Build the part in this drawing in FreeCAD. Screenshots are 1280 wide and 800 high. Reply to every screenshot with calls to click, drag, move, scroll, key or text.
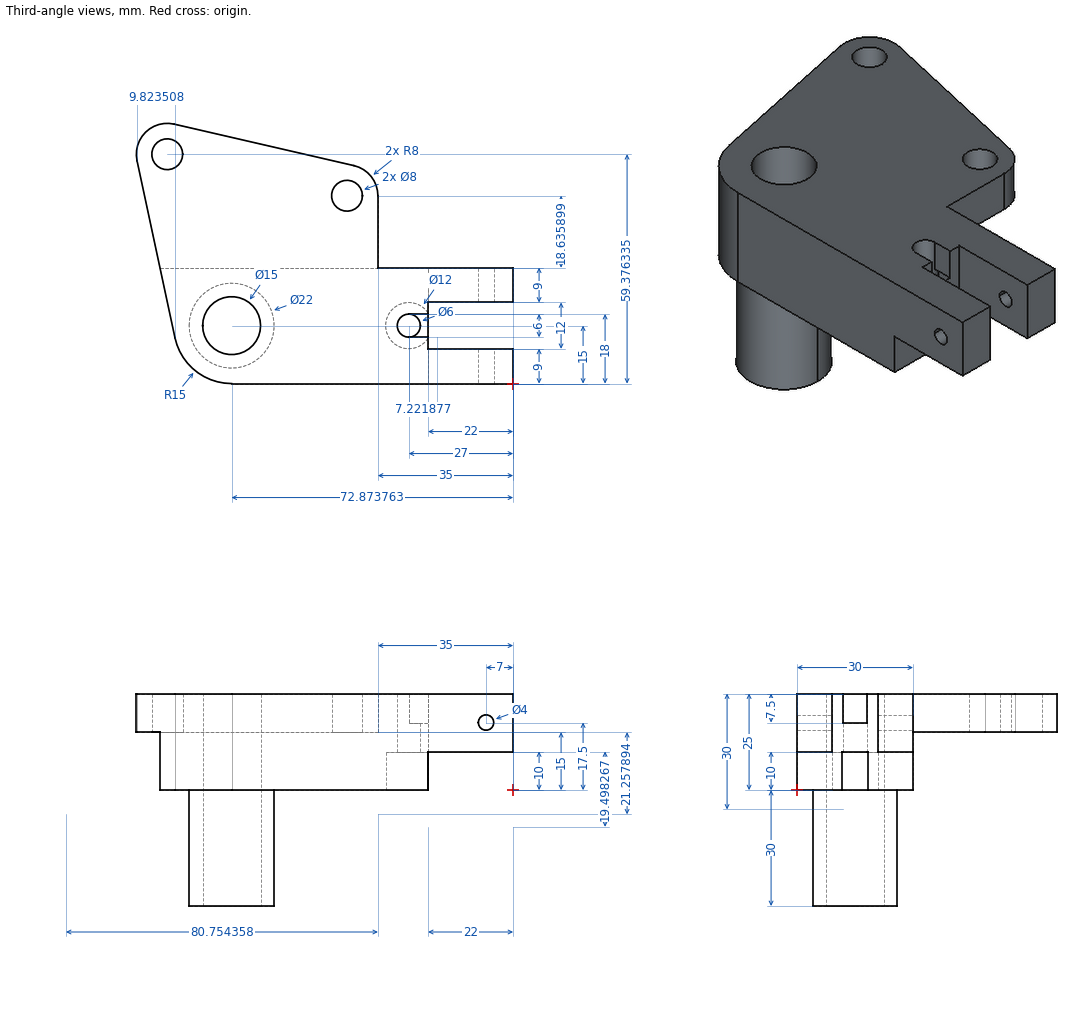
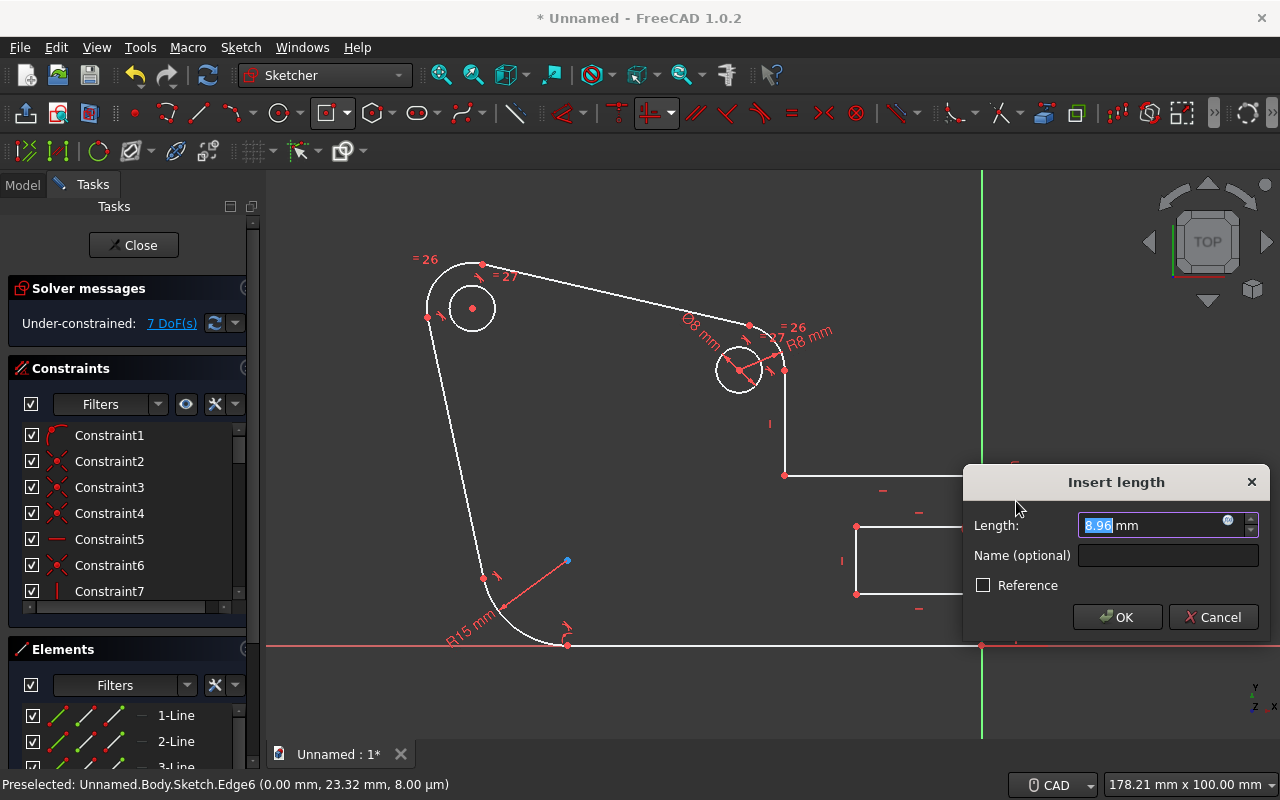
text(9)
key(Return)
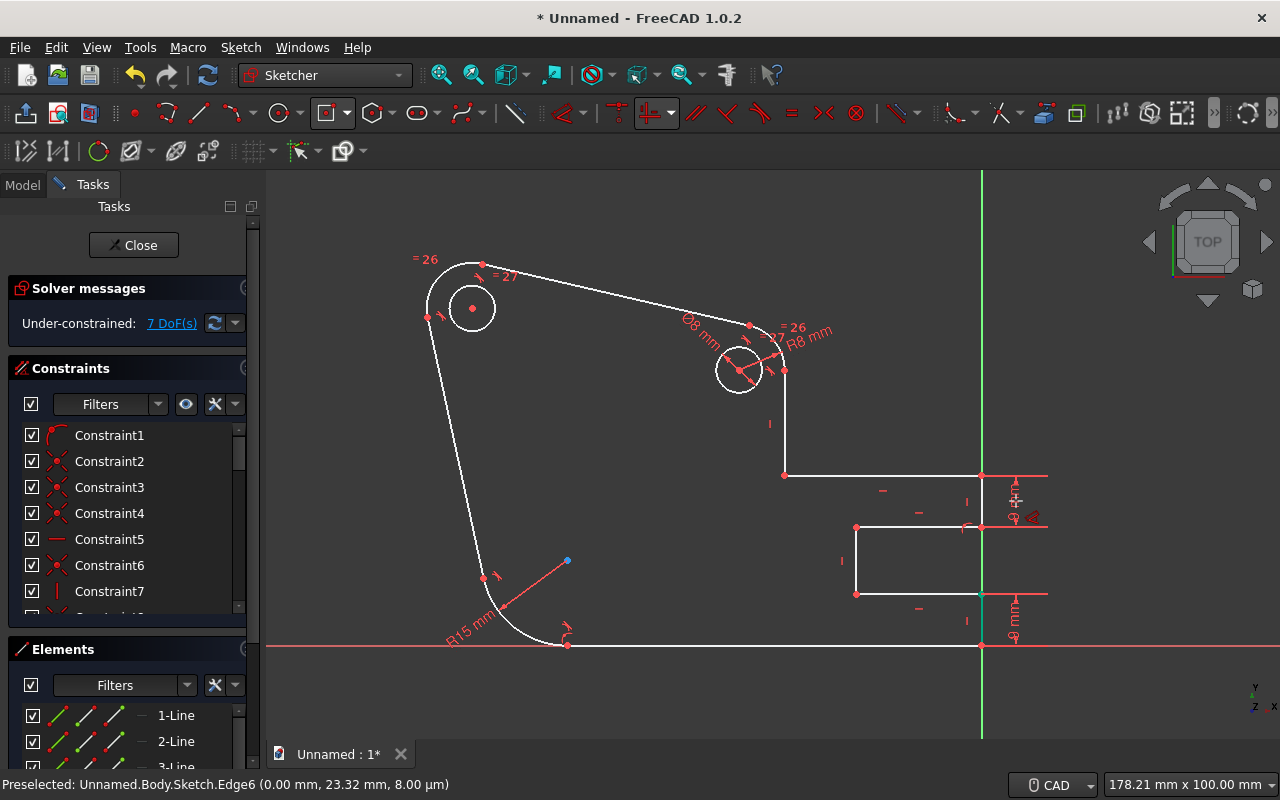
click(944, 594)
click(919, 628)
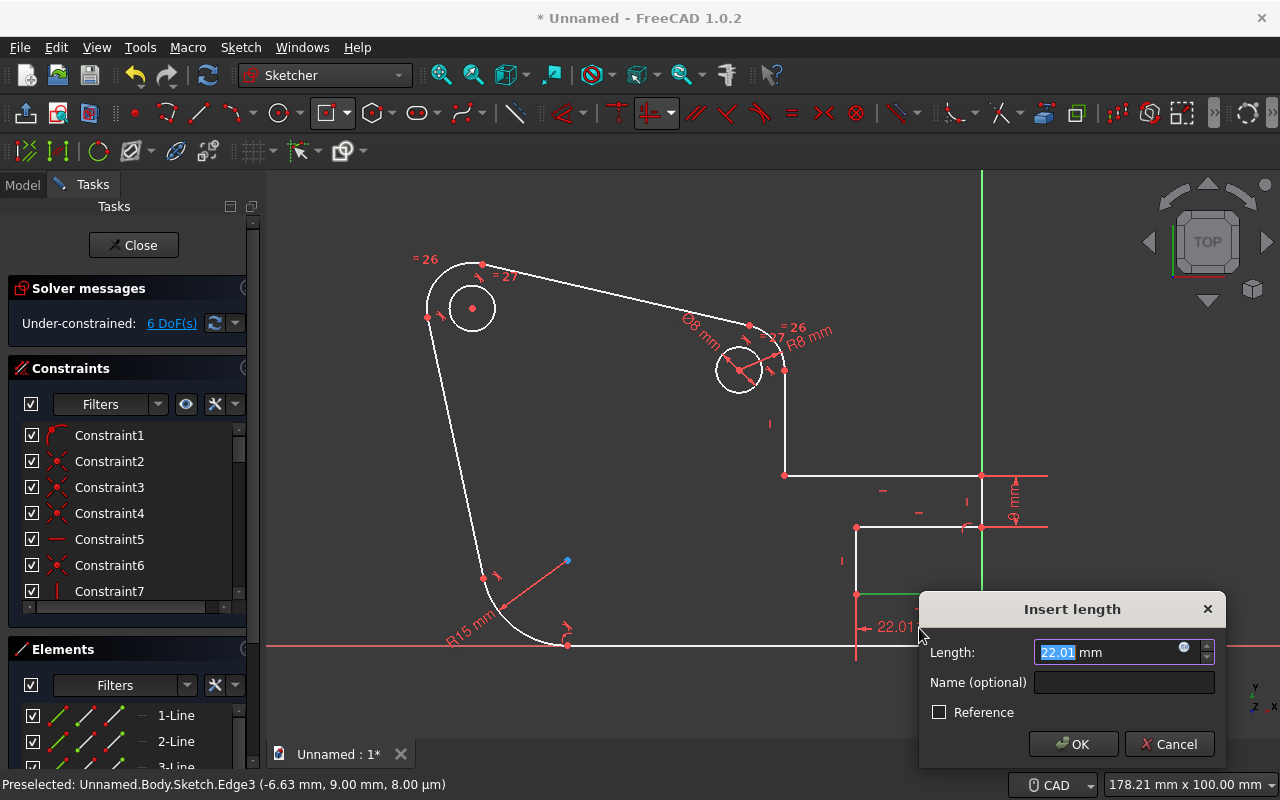
text(22)
key(Return)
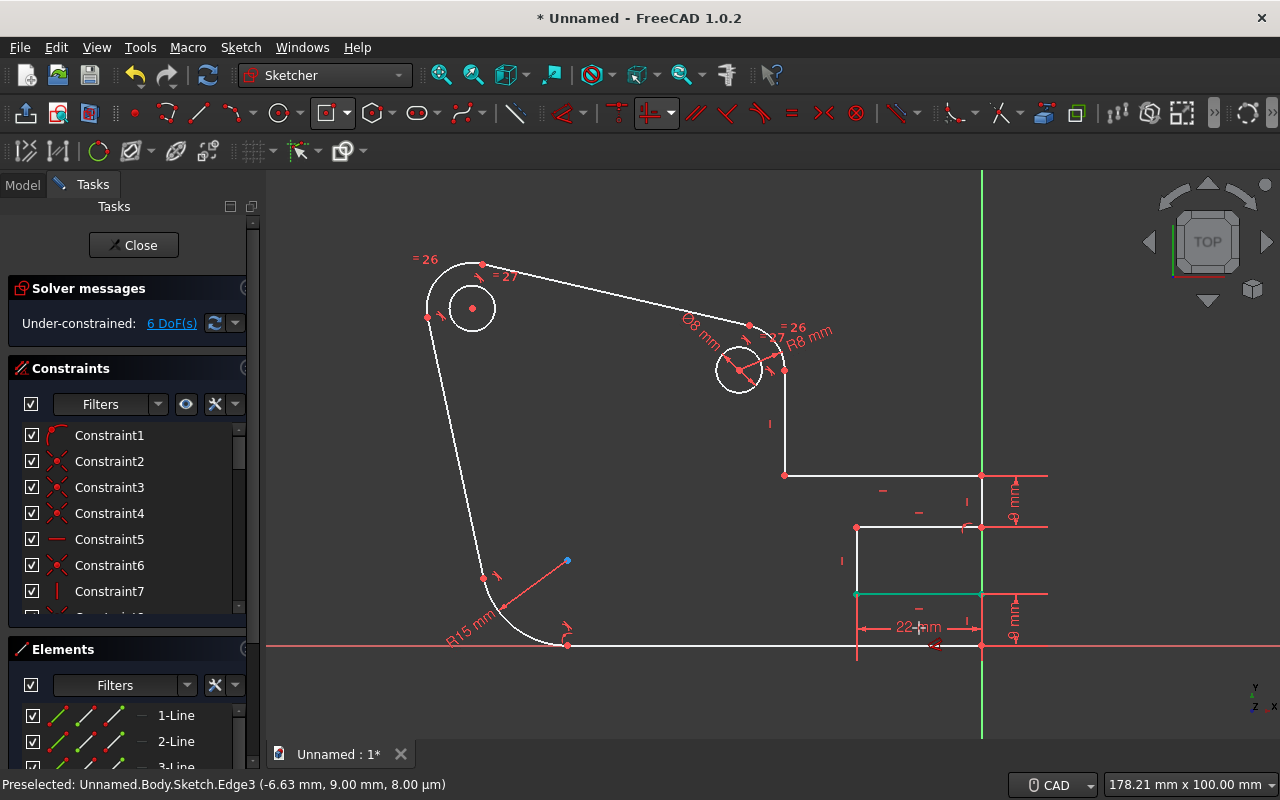
click(857, 574)
click(891, 561)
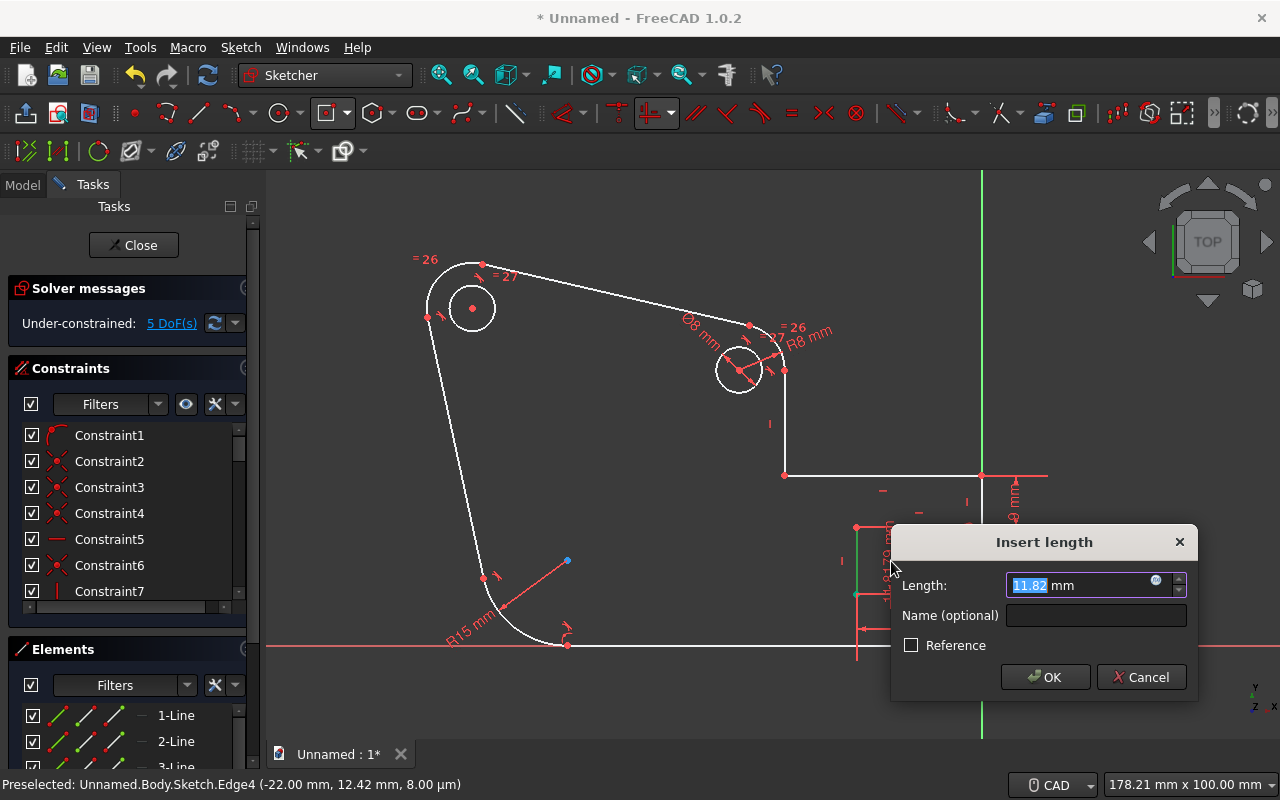
text(12)
key(Return)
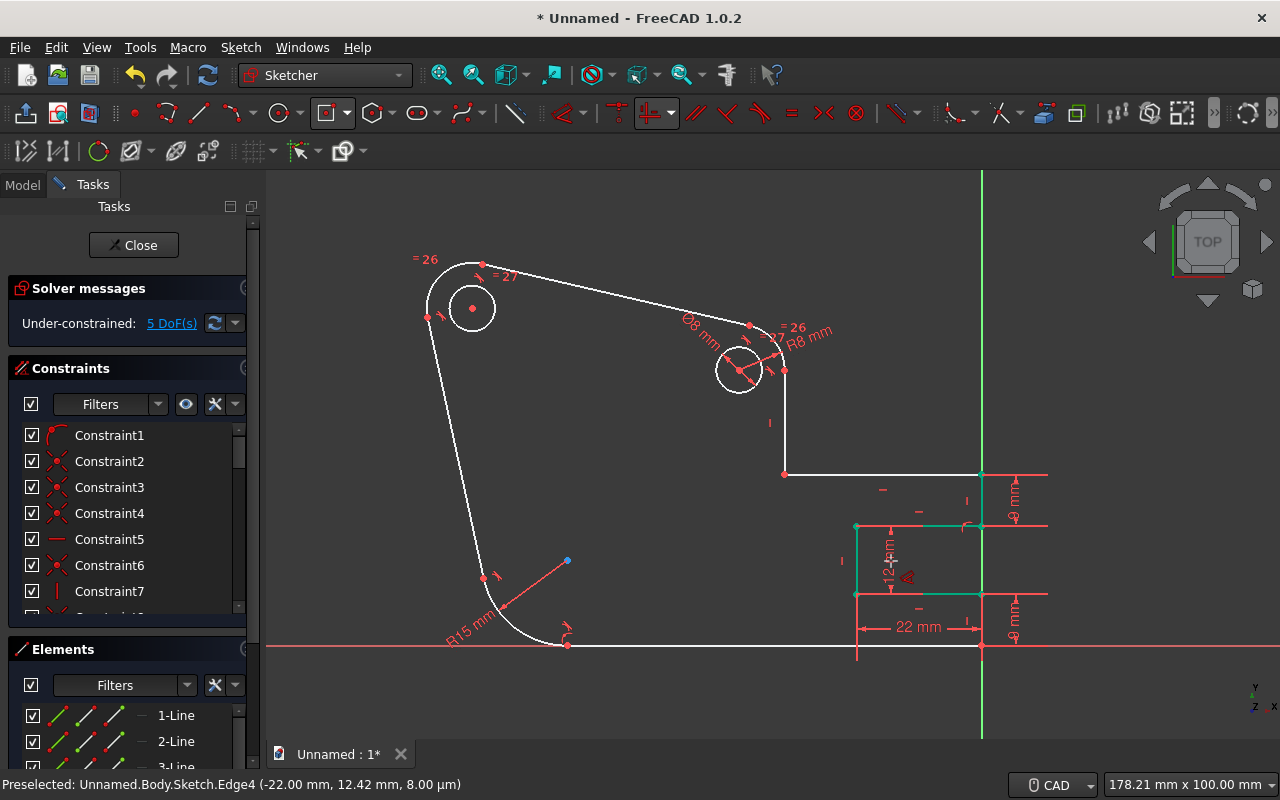
click(923, 475)
click(883, 509)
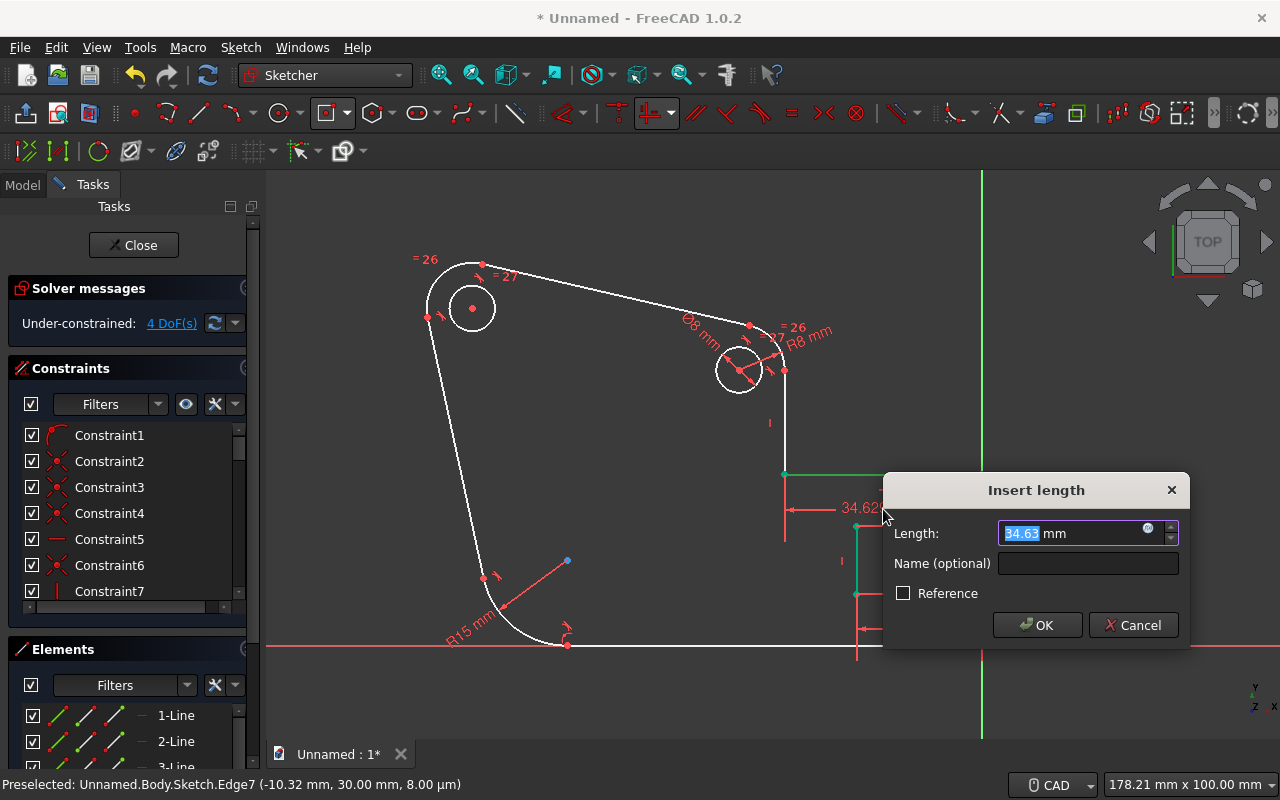
text(35)
key(Return)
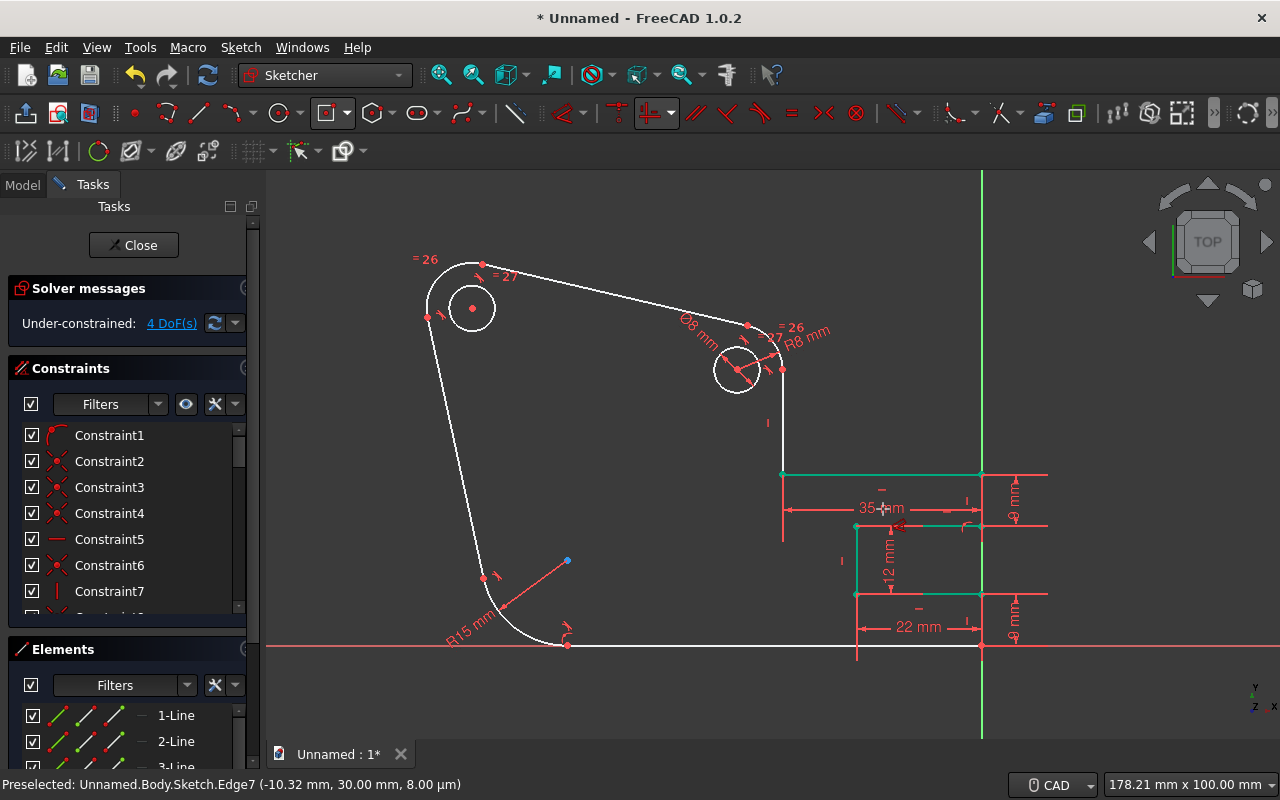
click(691, 646)
click(774, 680)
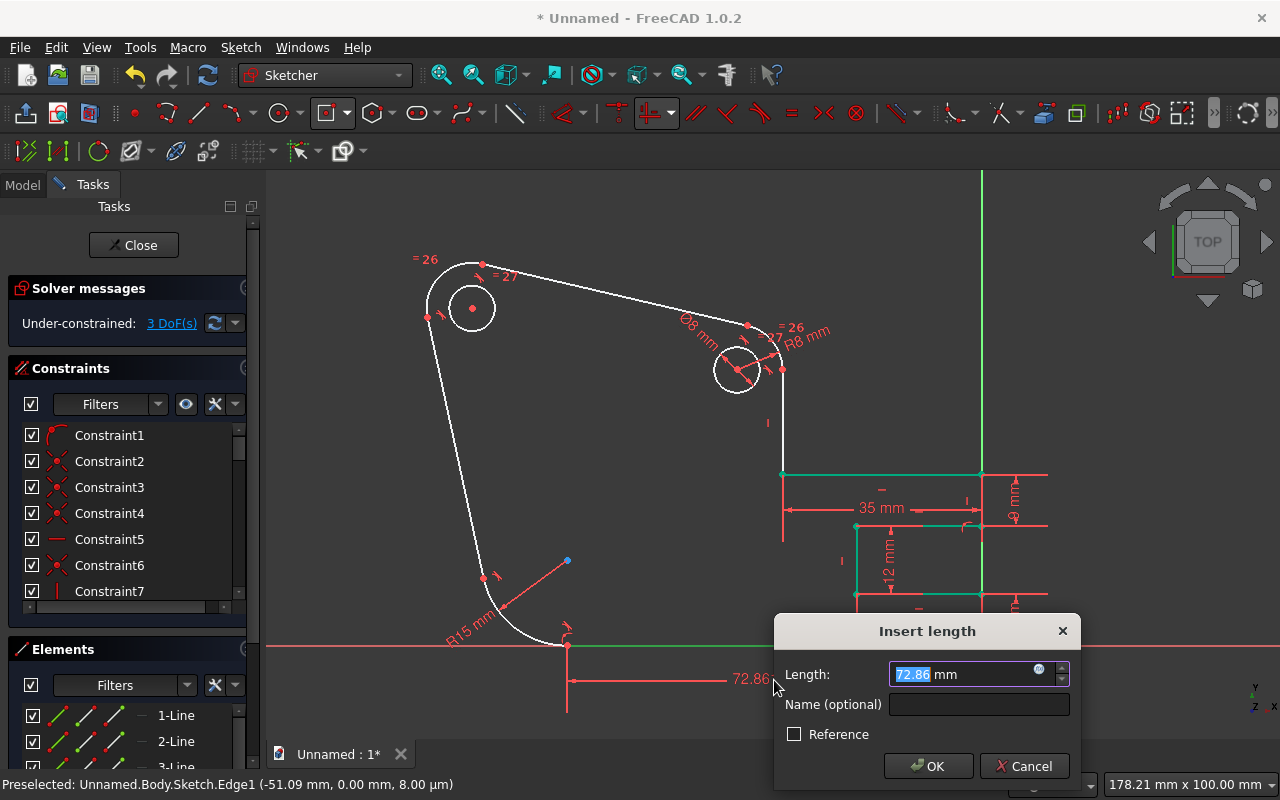
text(72.873763)
key(Return)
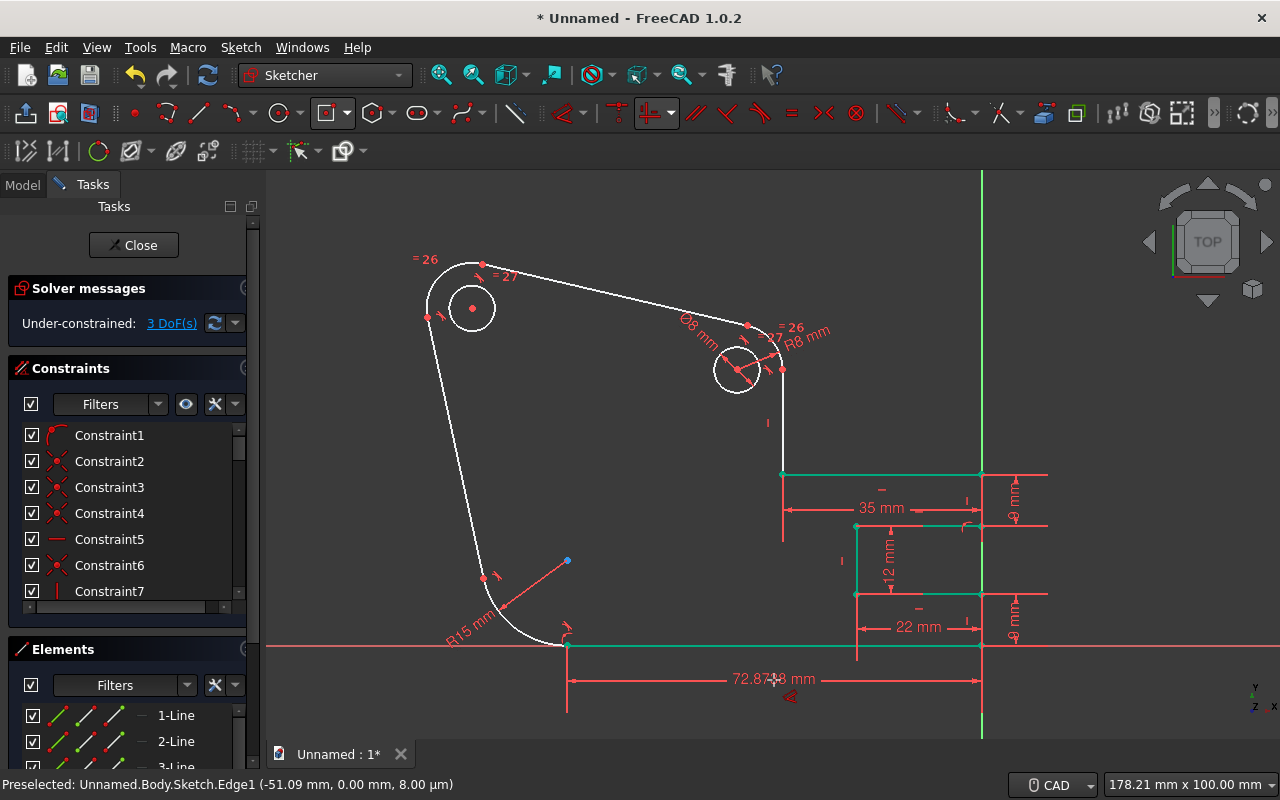
click(783, 443)
click(817, 422)